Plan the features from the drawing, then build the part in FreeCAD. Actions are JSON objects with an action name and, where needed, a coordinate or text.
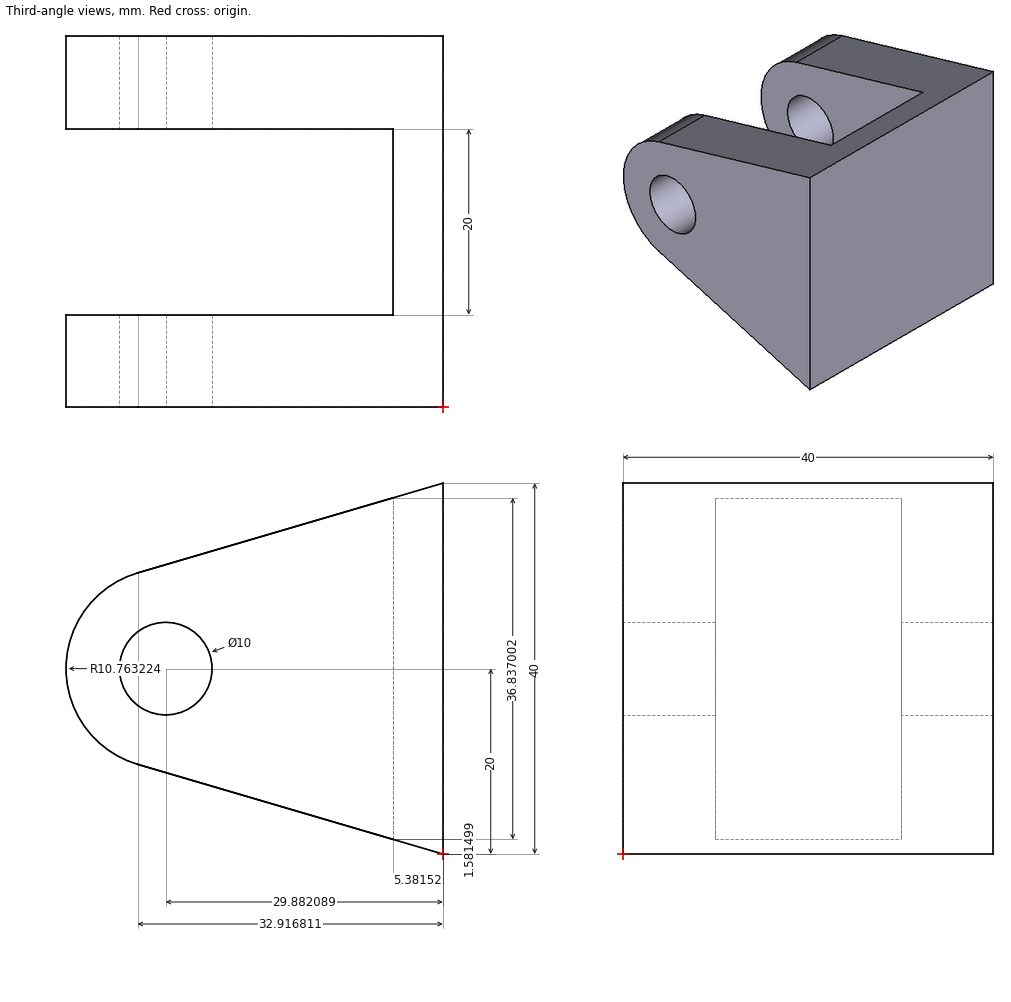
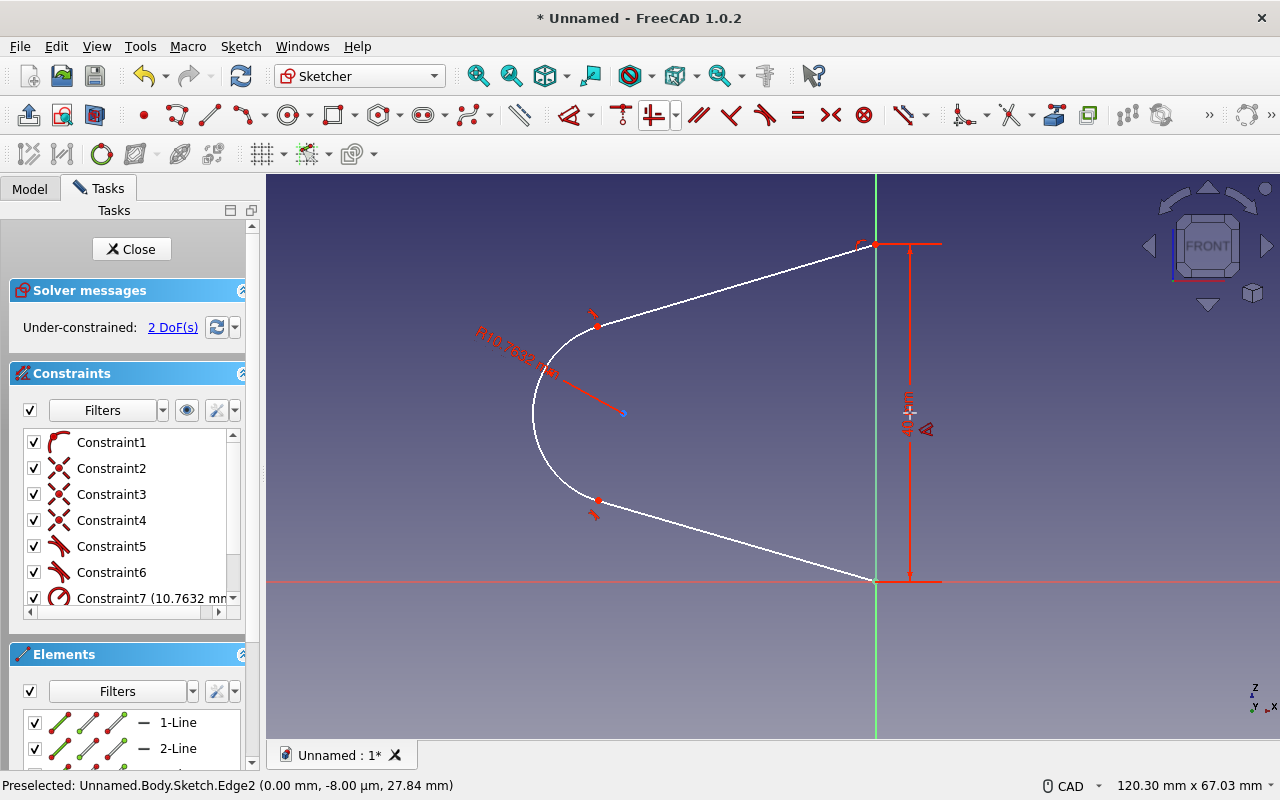
{"action": "left_click", "coordinate": [624, 414]}
{"action": "left_click", "coordinate": [910, 498]}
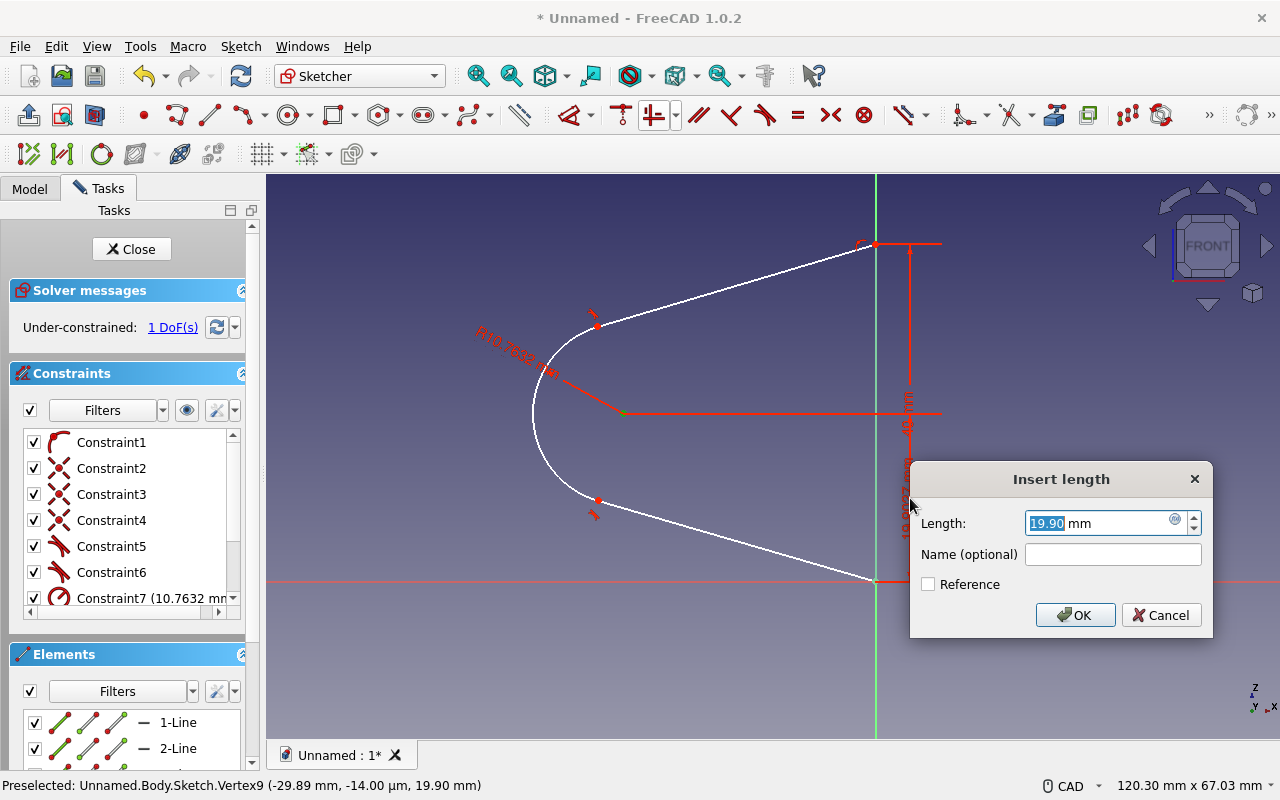
{"action": "type", "text": "20"}
{"action": "key", "text": "Return"}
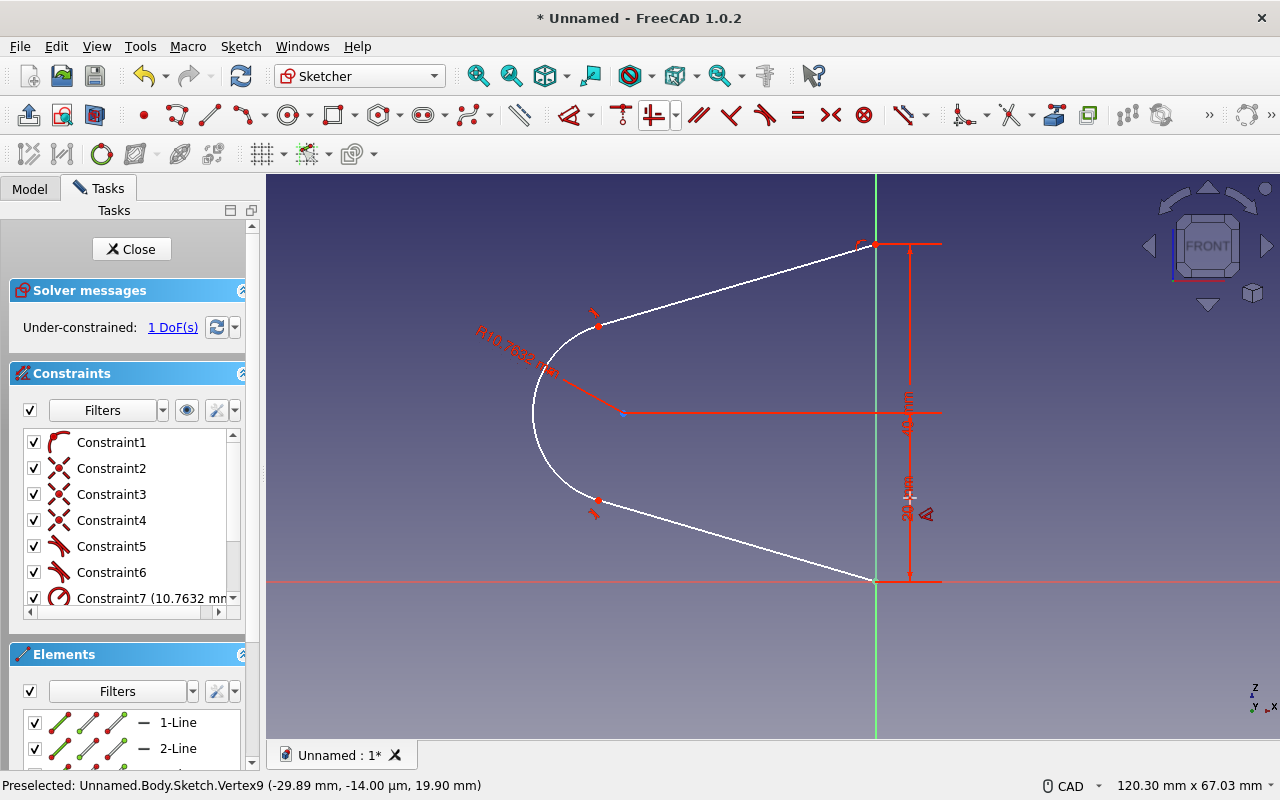
{"action": "left_click", "coordinate": [598, 326]}
{"action": "left_click", "coordinate": [737, 616]}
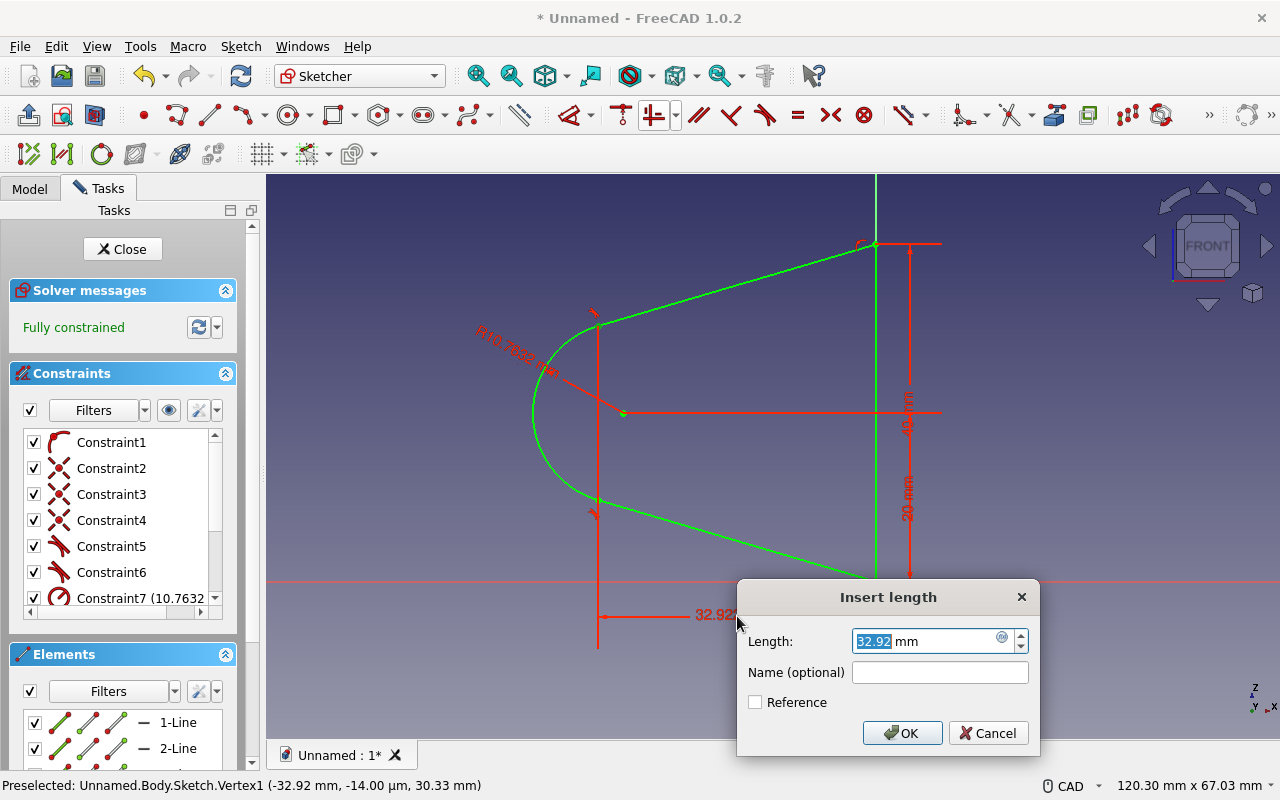
{"action": "type", "text": "32.916811"}
{"action": "key", "text": "Return"}
{"action": "key", "text": "Escape"}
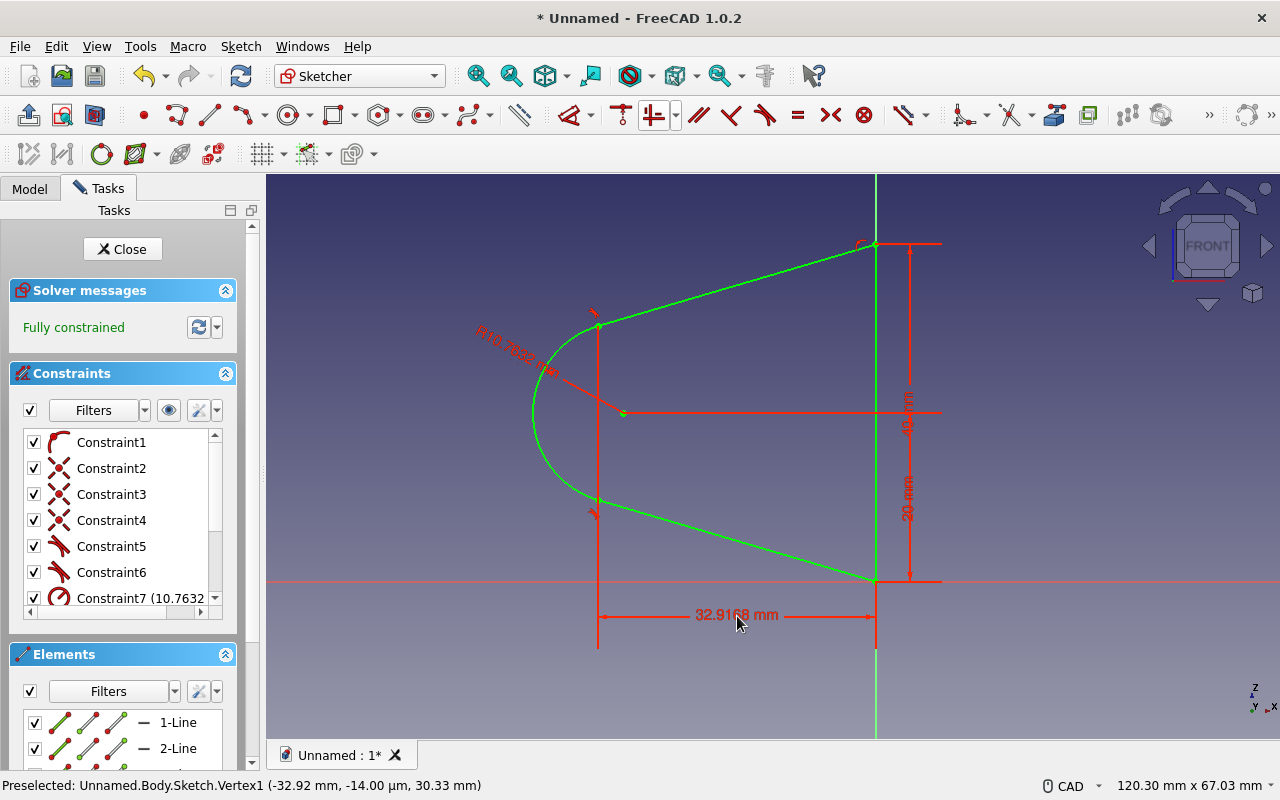
{"action": "left_click", "coordinate": [123, 249]}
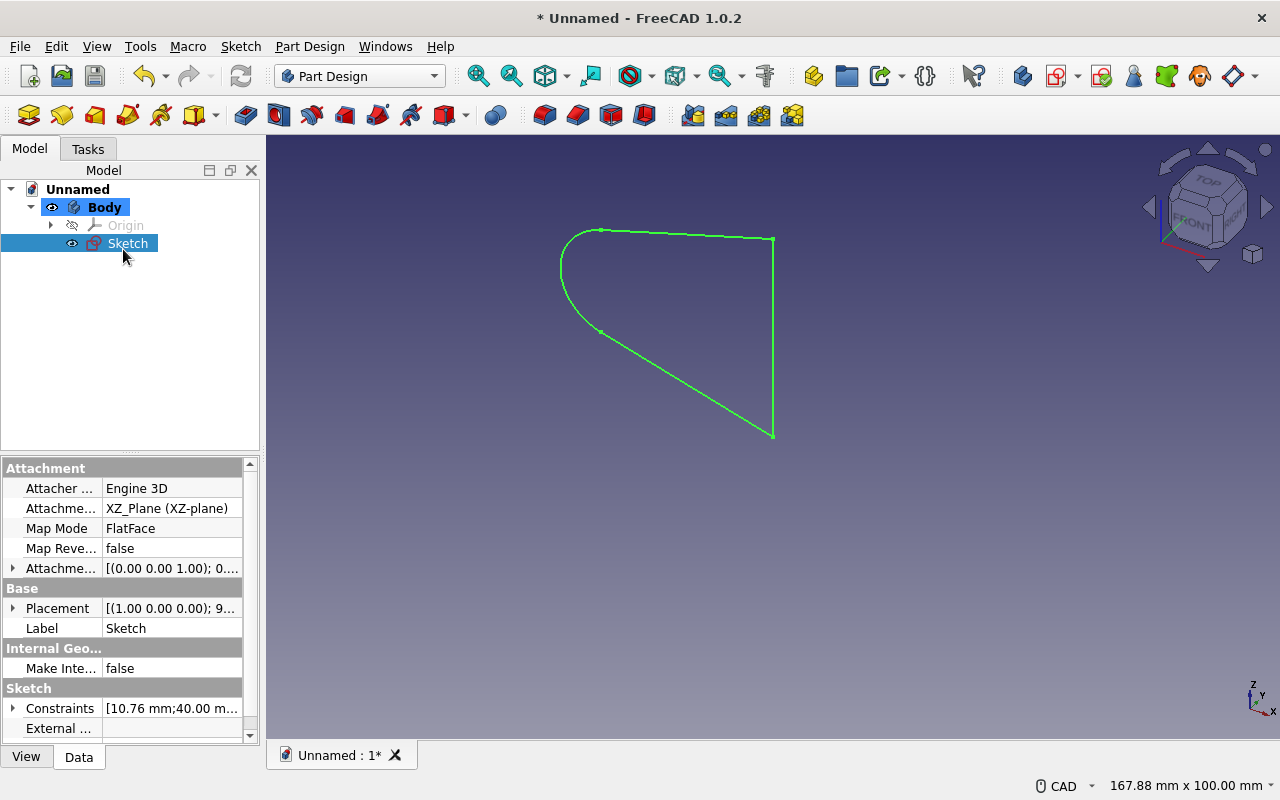
{"action": "left_click", "coordinate": [29, 116]}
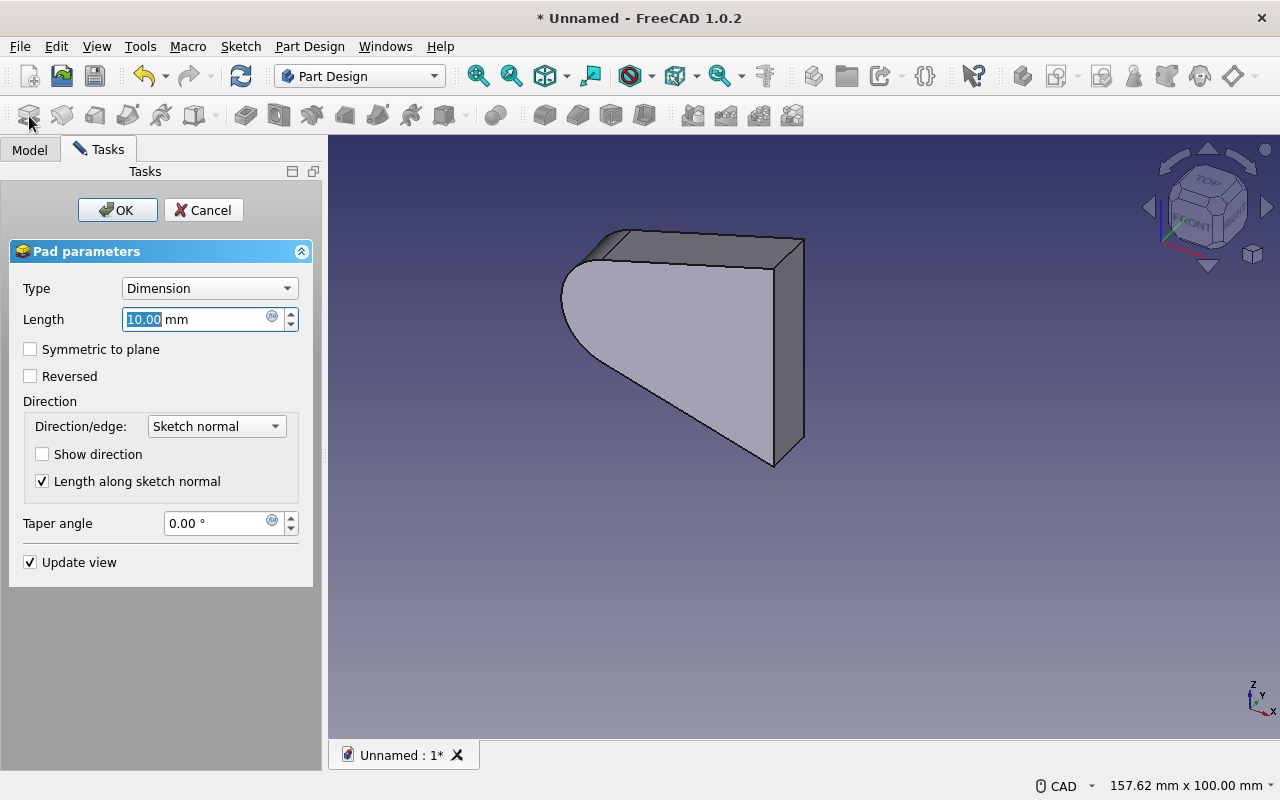
{"action": "type", "text": "40"}
{"action": "key", "text": "Tab"}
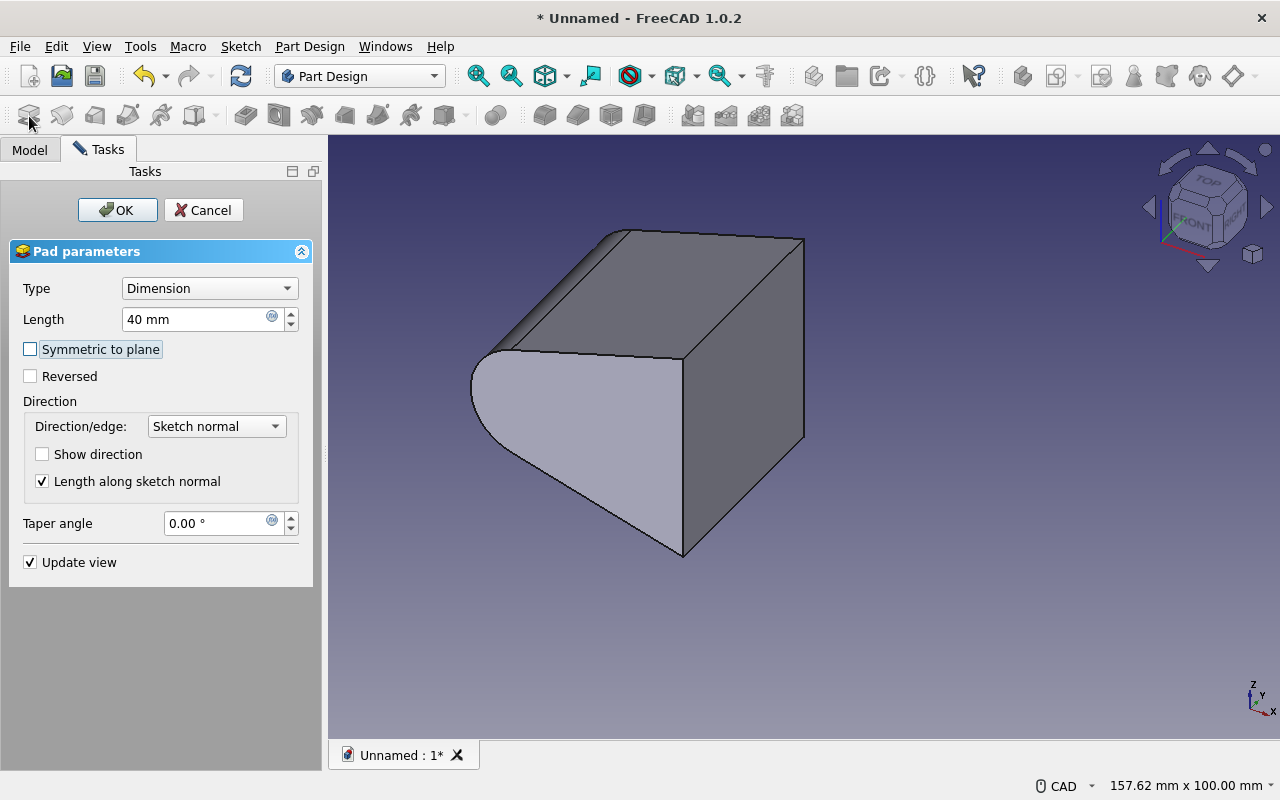
{"action": "left_click", "coordinate": [31, 376]}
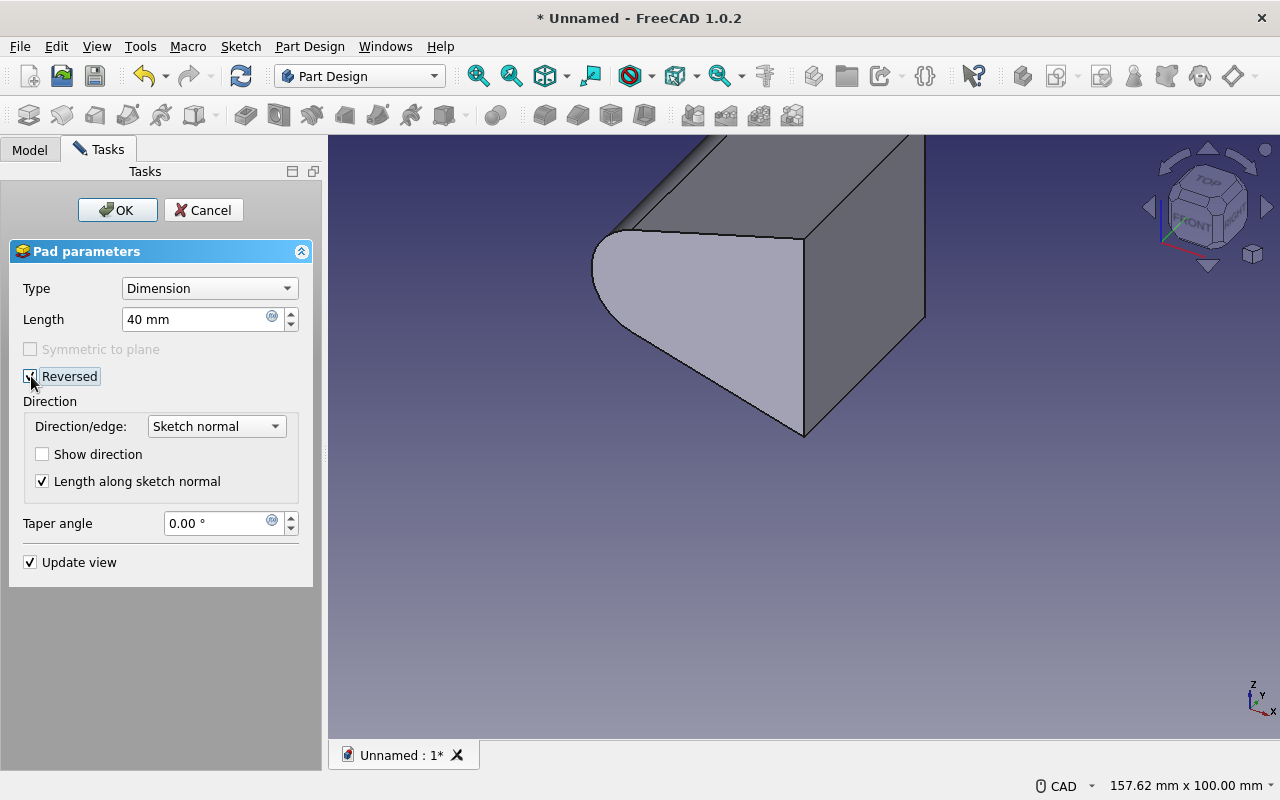
{"action": "left_click", "coordinate": [118, 210]}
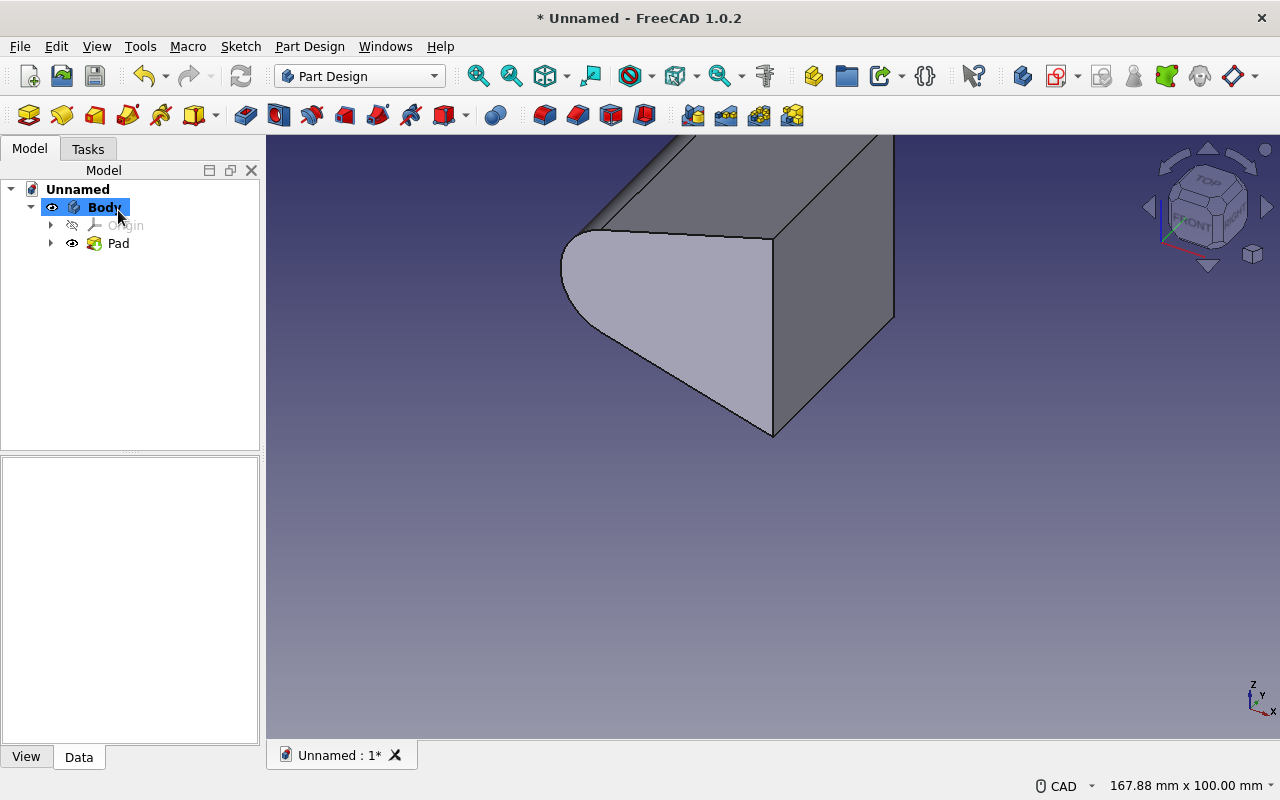
{"action": "left_click", "coordinate": [479, 76]}